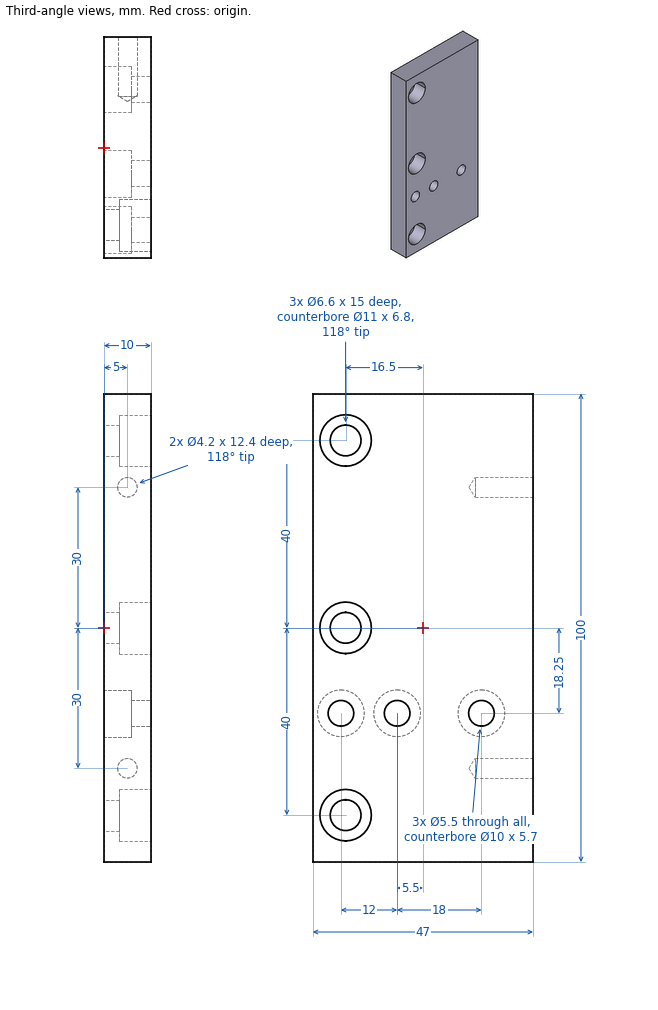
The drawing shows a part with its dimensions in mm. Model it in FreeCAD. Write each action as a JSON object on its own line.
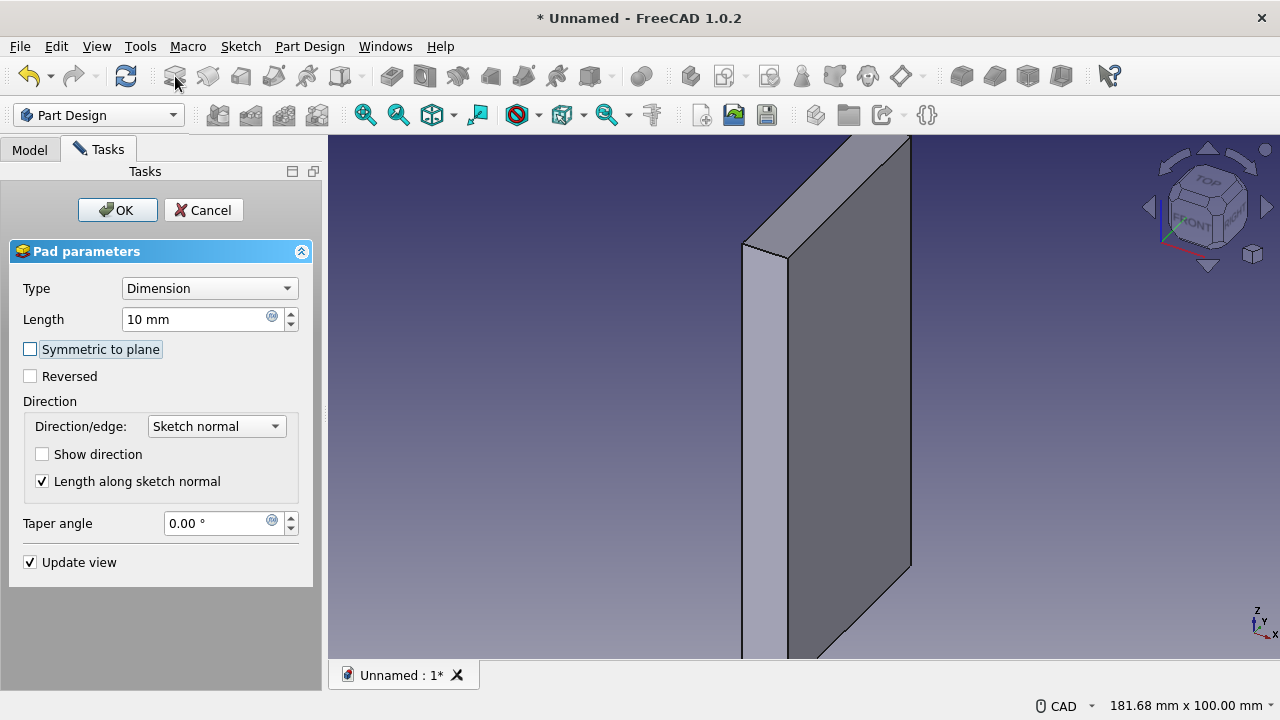
{"action": "left_click", "coordinate": [118, 210]}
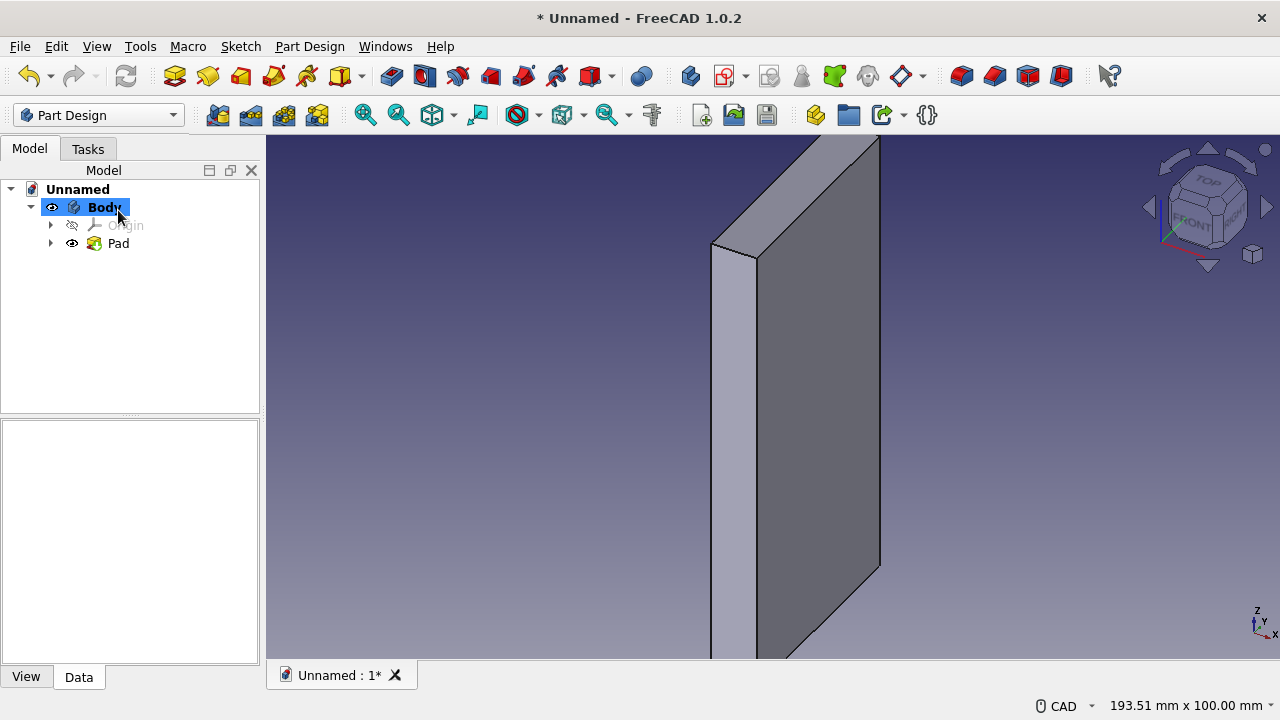
{"action": "left_click", "coordinate": [366, 116]}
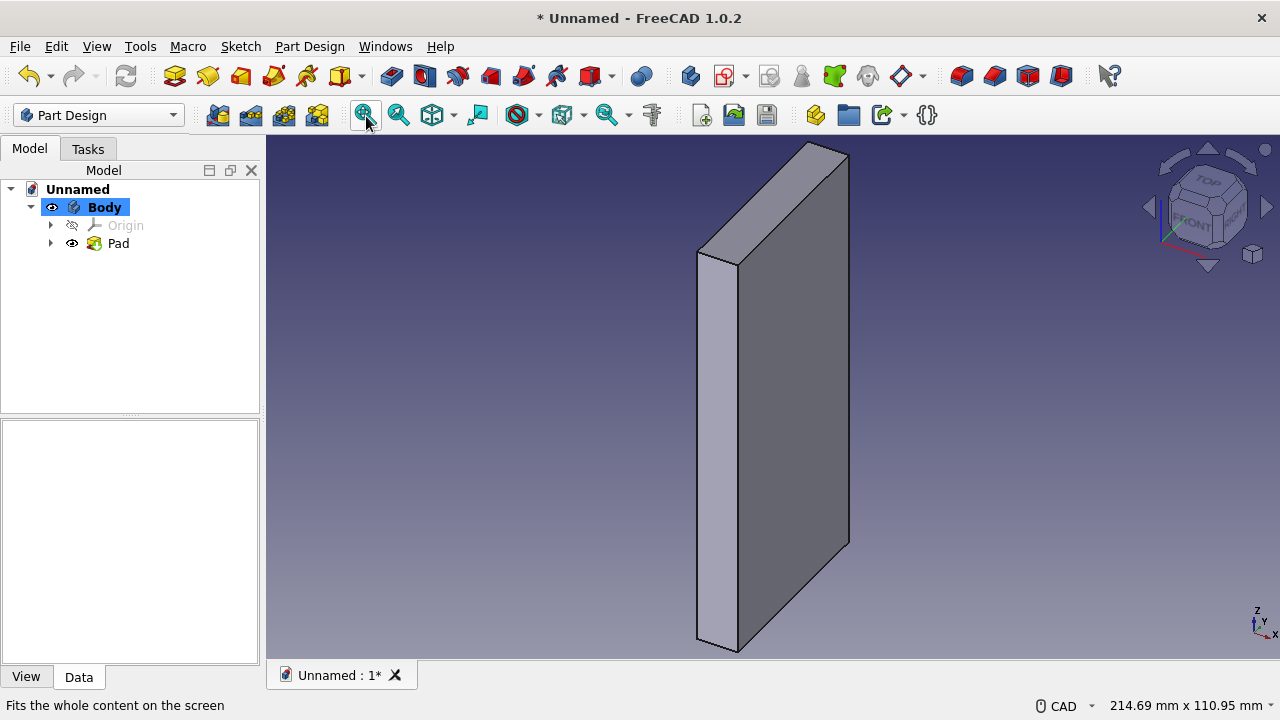
{"action": "left_click", "coordinate": [793, 403]}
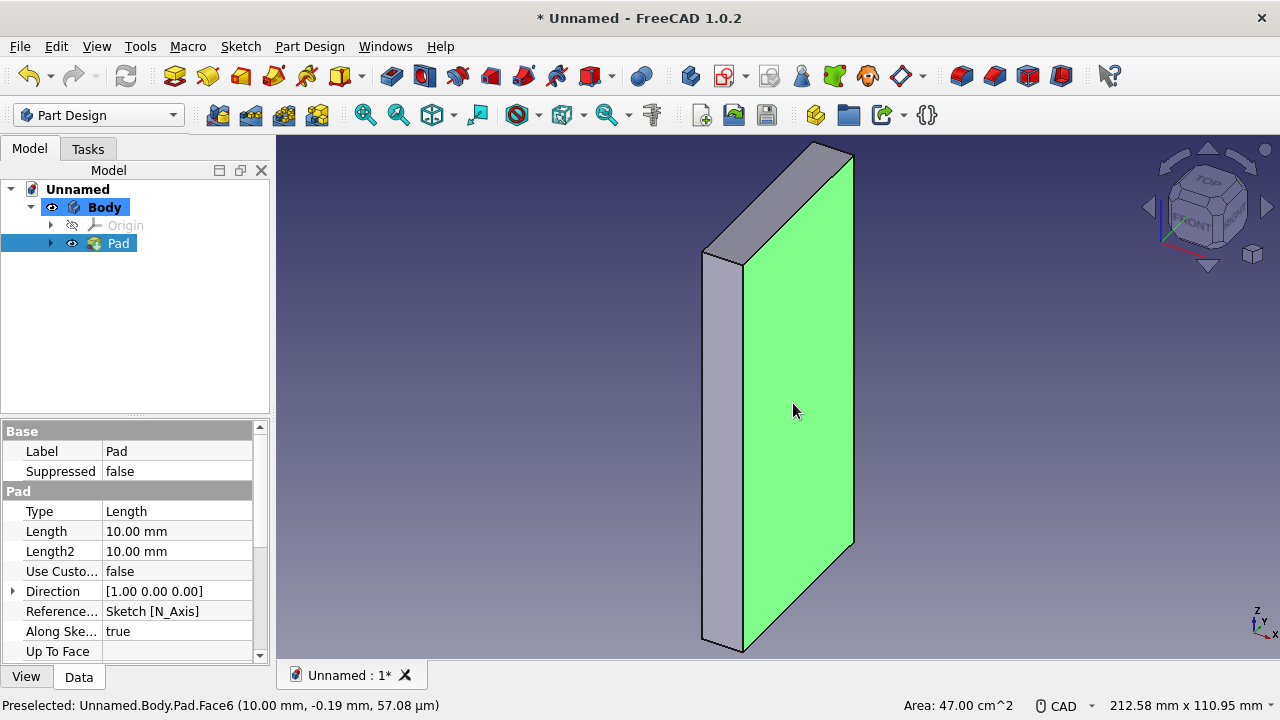
{"action": "left_click", "coordinate": [724, 76]}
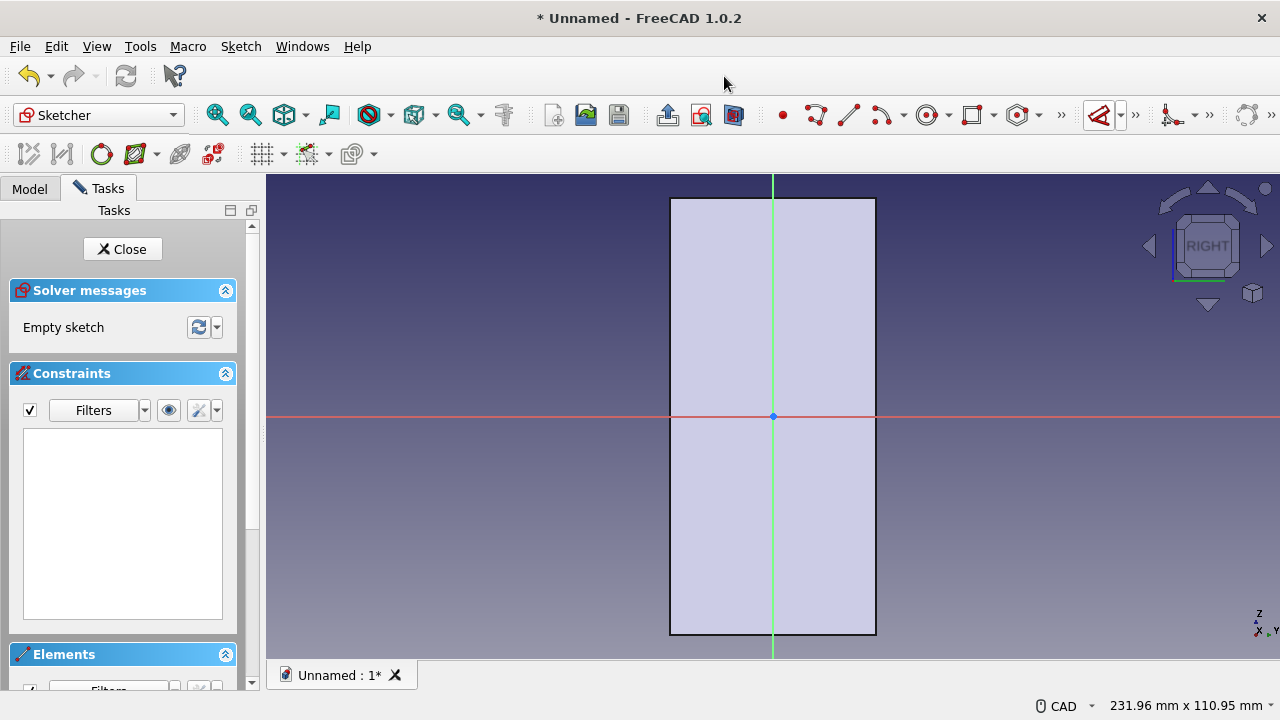
{"action": "left_click", "coordinate": [926, 116]}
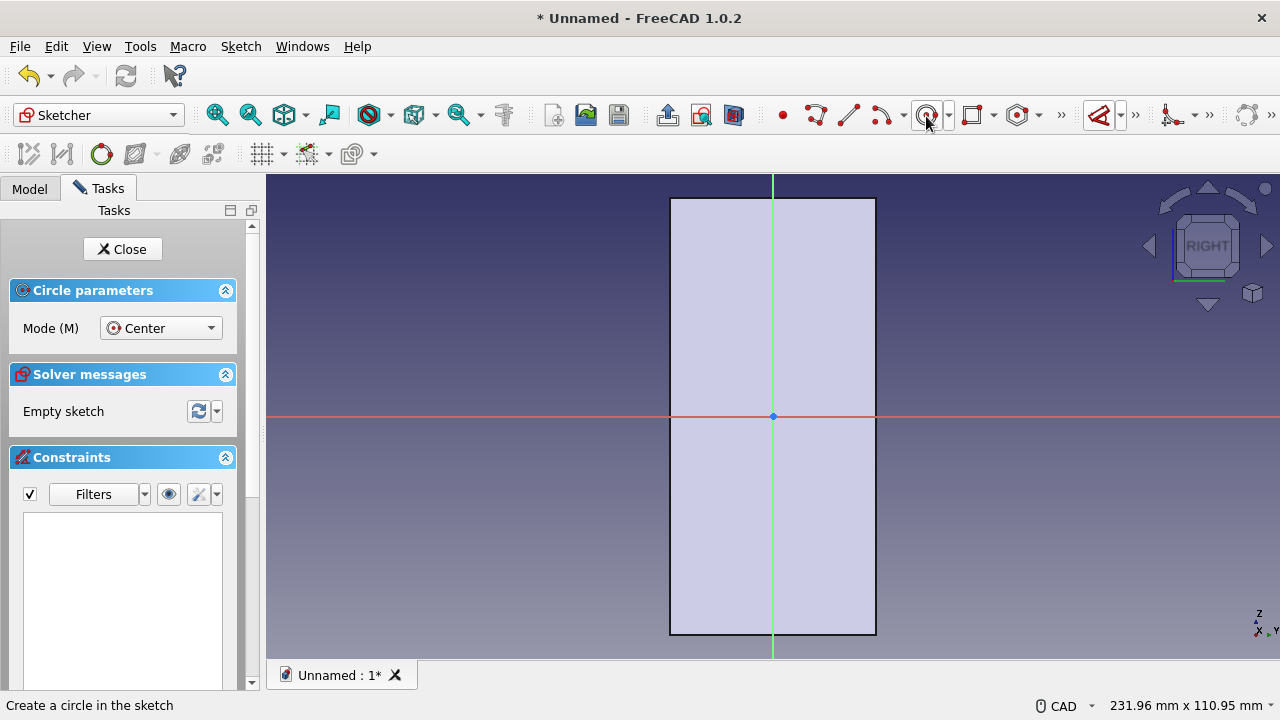
{"action": "scroll", "coordinate": [701, 242], "scroll_direction": "up", "scroll_amount": 3}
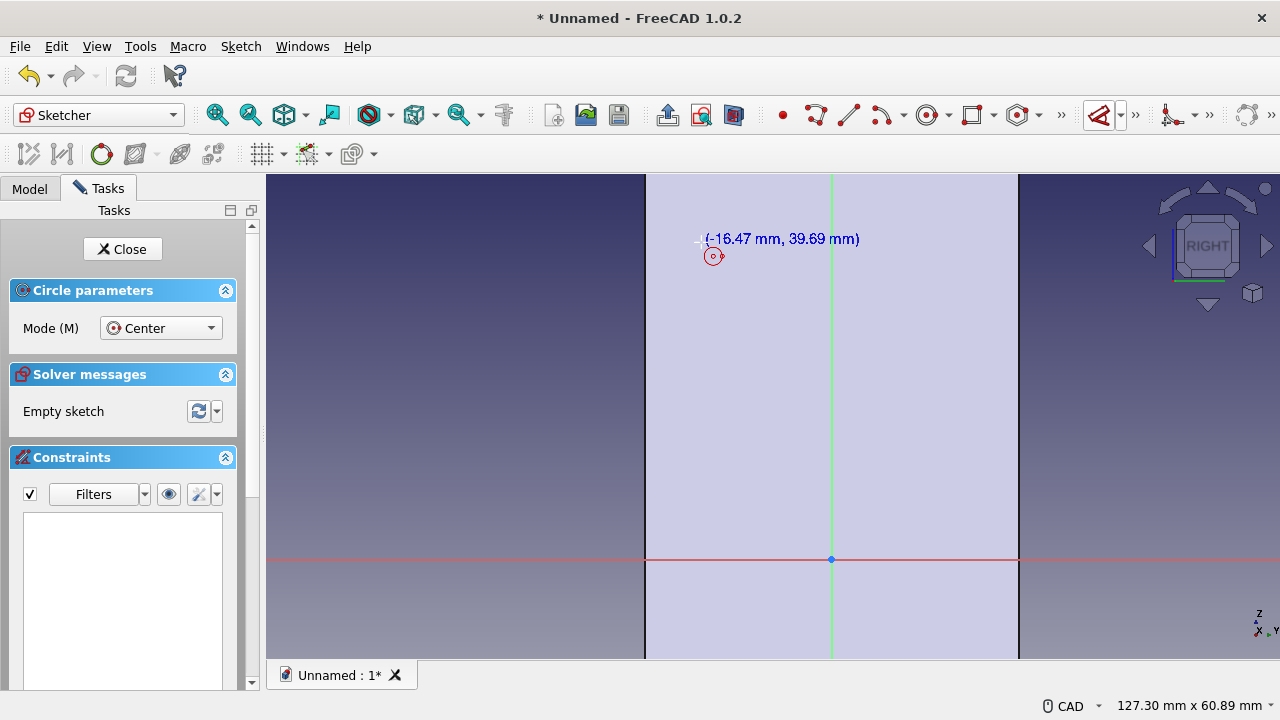
{"action": "left_click", "coordinate": [700, 241]}
{"action": "mouse_move", "coordinate": [719, 223]}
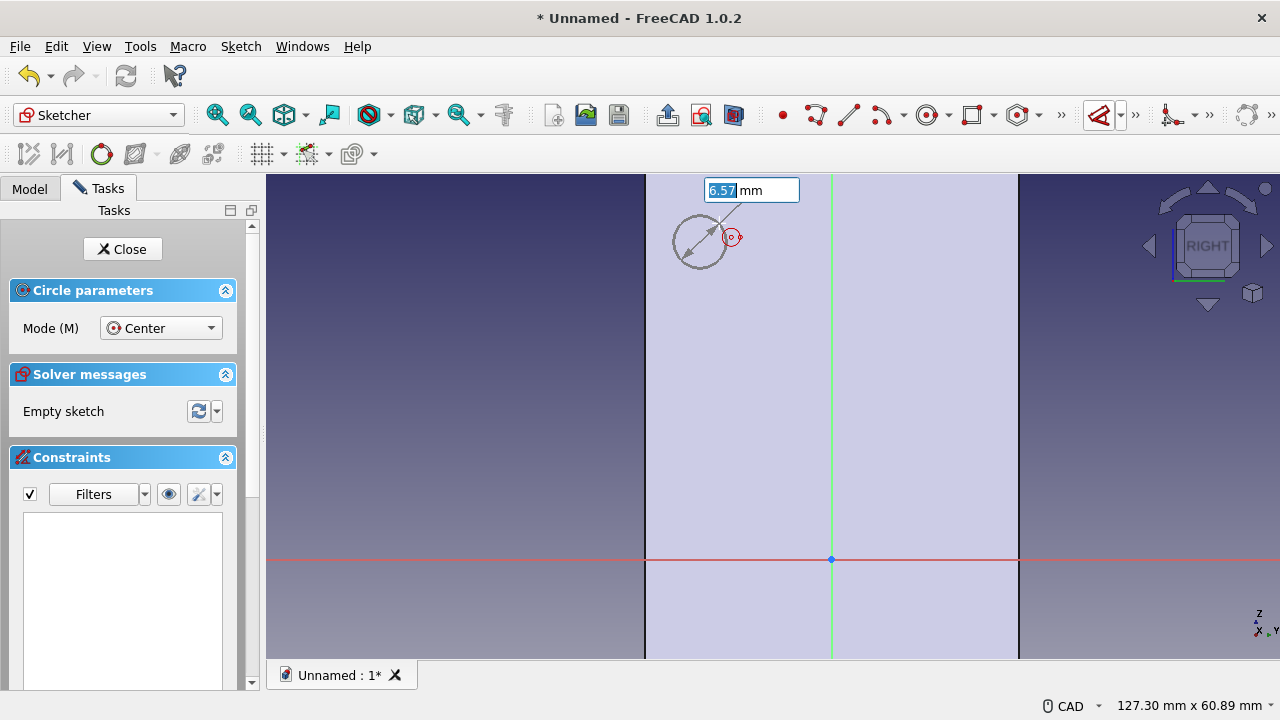
{"action": "type", "text": "6.6"}
{"action": "key", "text": "Return"}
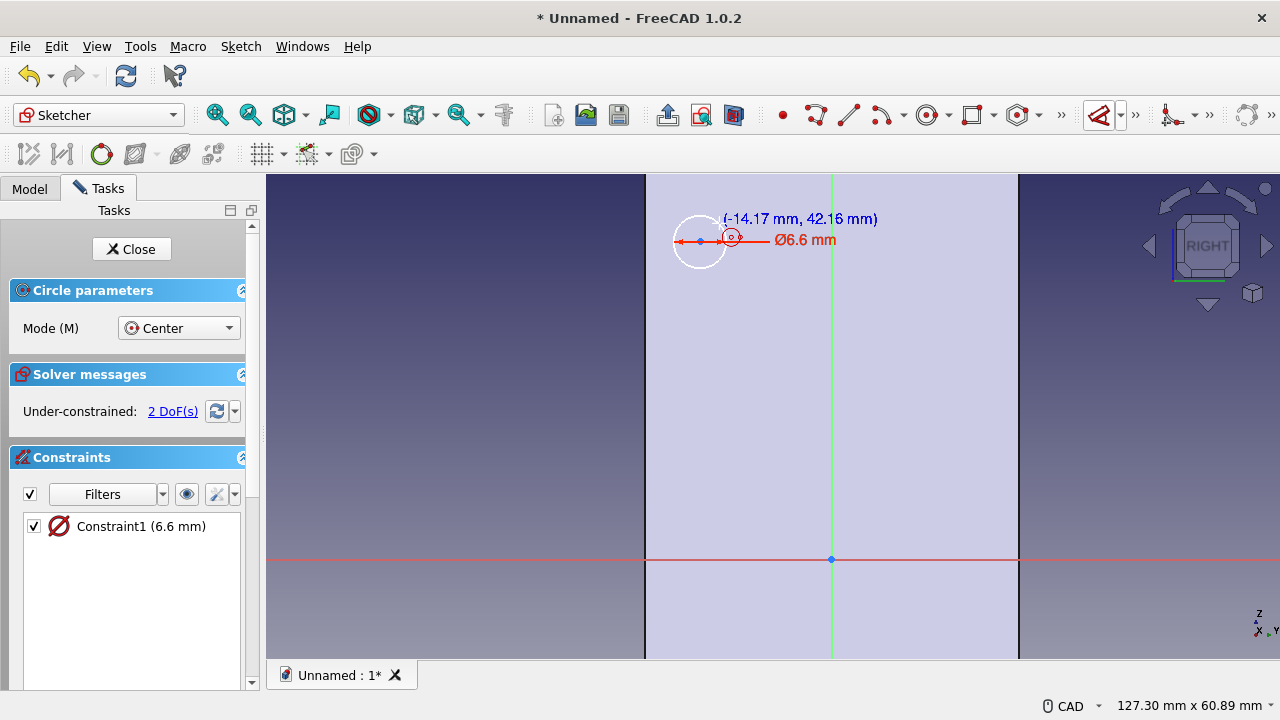
{"action": "left_click", "coordinate": [700, 560]}
{"action": "mouse_move", "coordinate": [719, 541]}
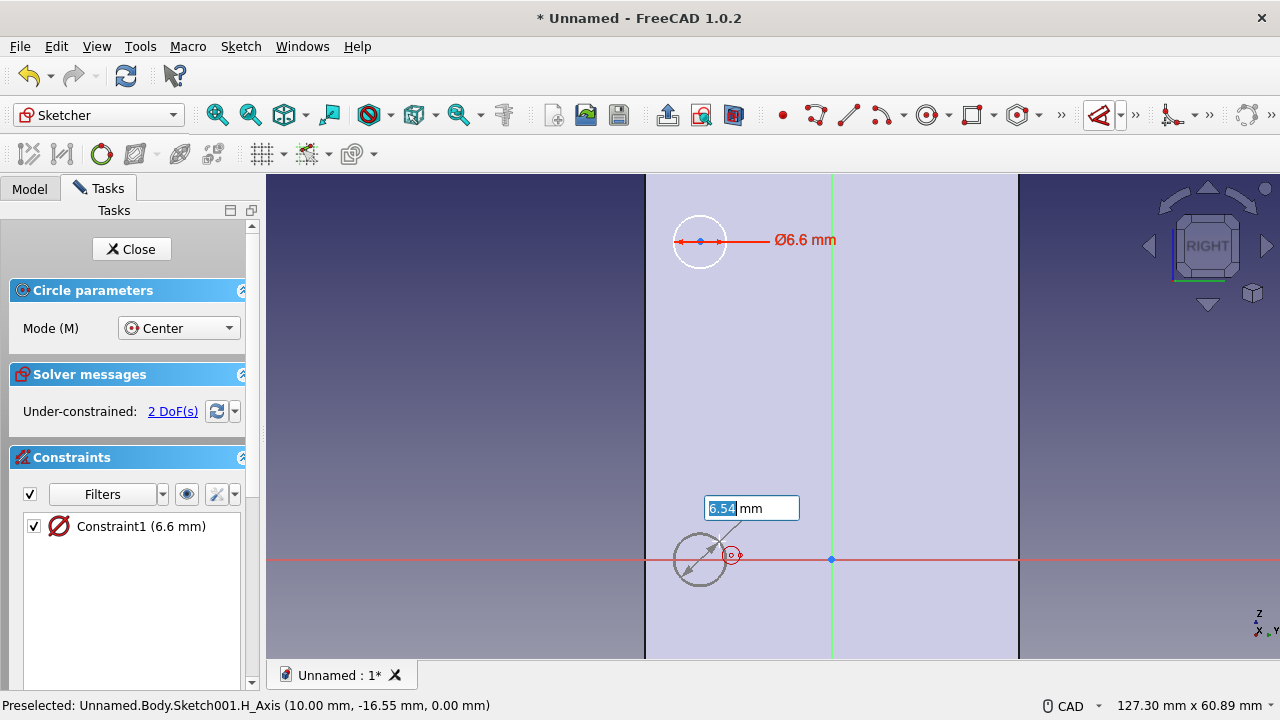
{"action": "type", "text": "6.6"}
{"action": "key", "text": "Return"}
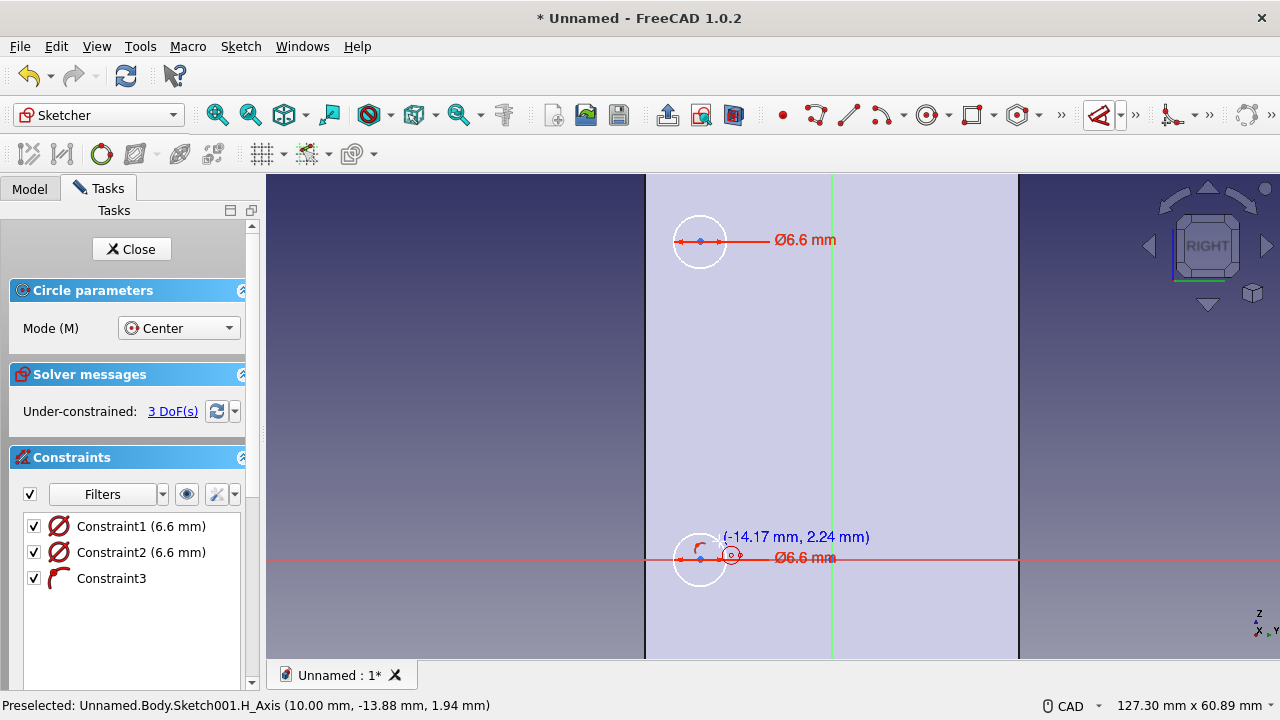
{"action": "scroll", "coordinate": [665, 300], "scroll_direction": "down", "scroll_amount": 4}